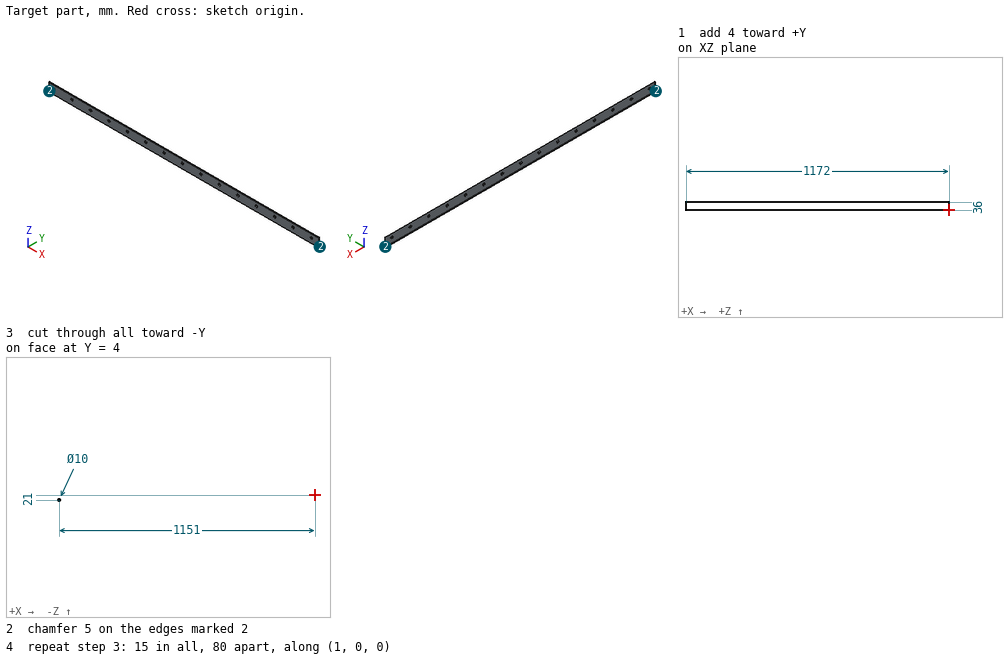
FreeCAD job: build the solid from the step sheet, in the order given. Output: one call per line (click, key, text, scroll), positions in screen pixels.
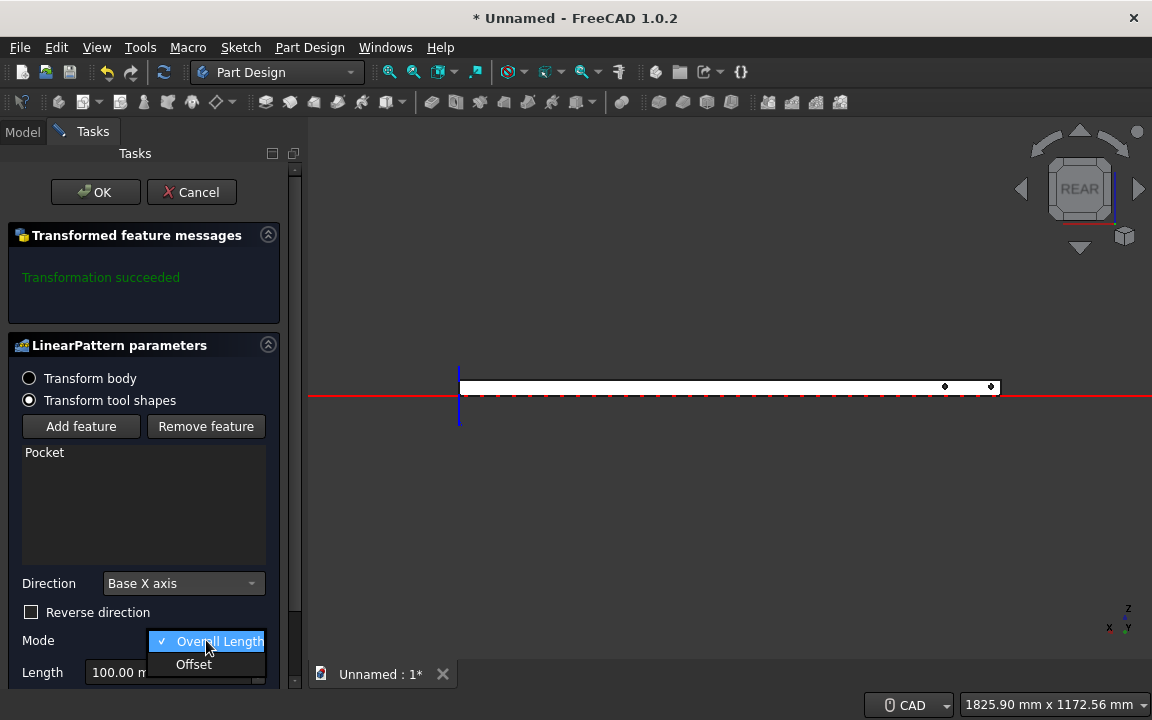
click(206, 664)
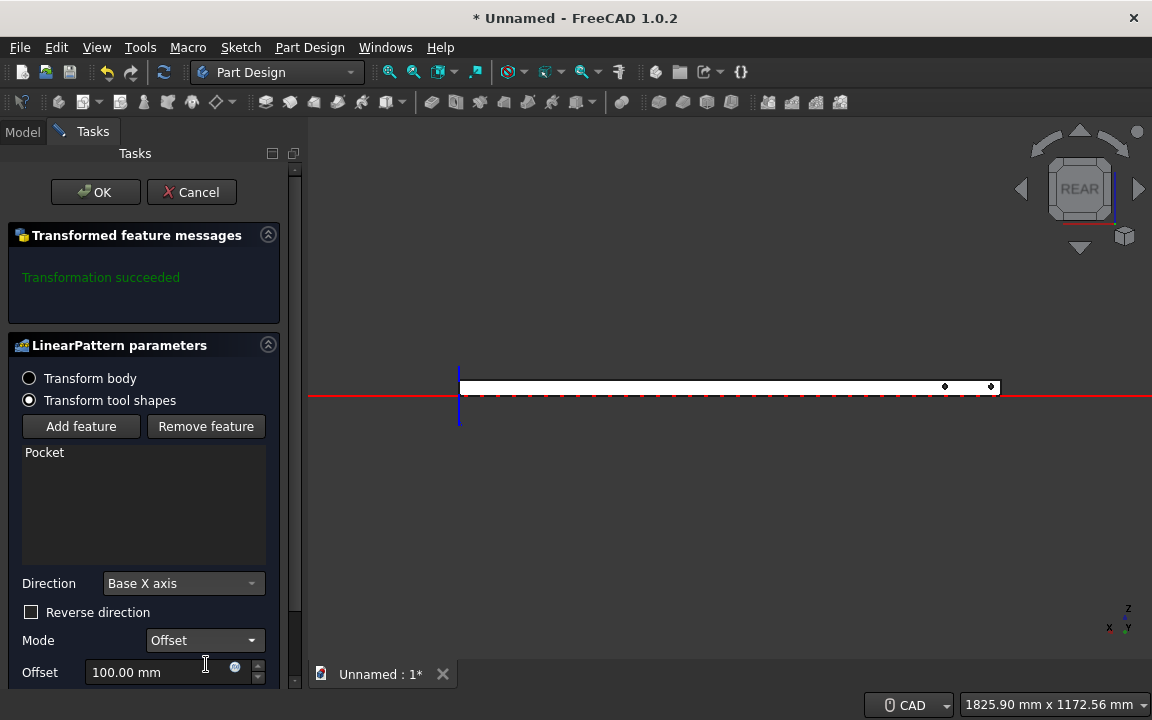
triple_click(168, 672)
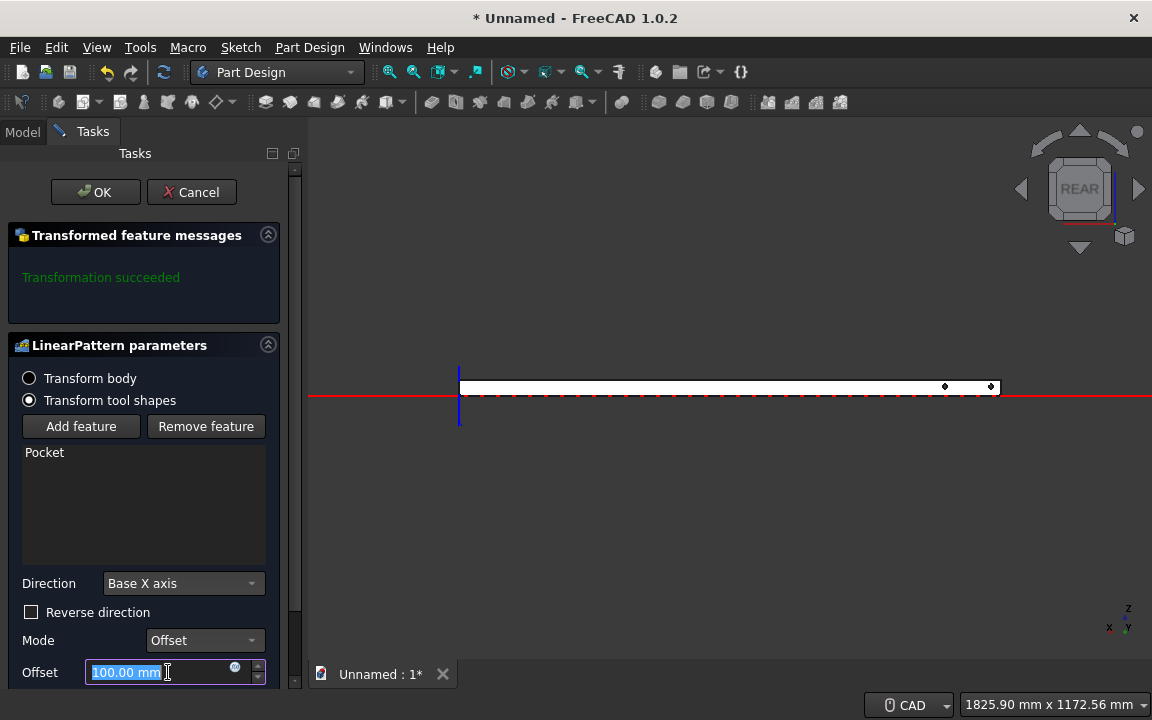
text(80)
key(Tab)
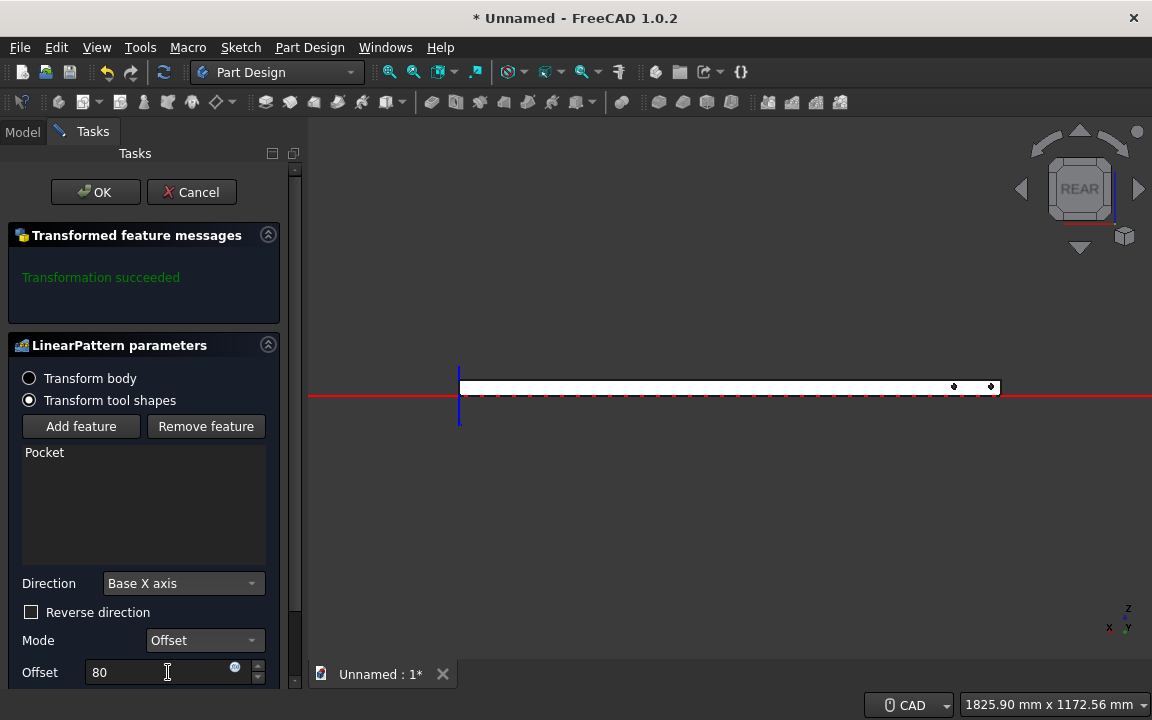
scroll(295, 426, down, 2)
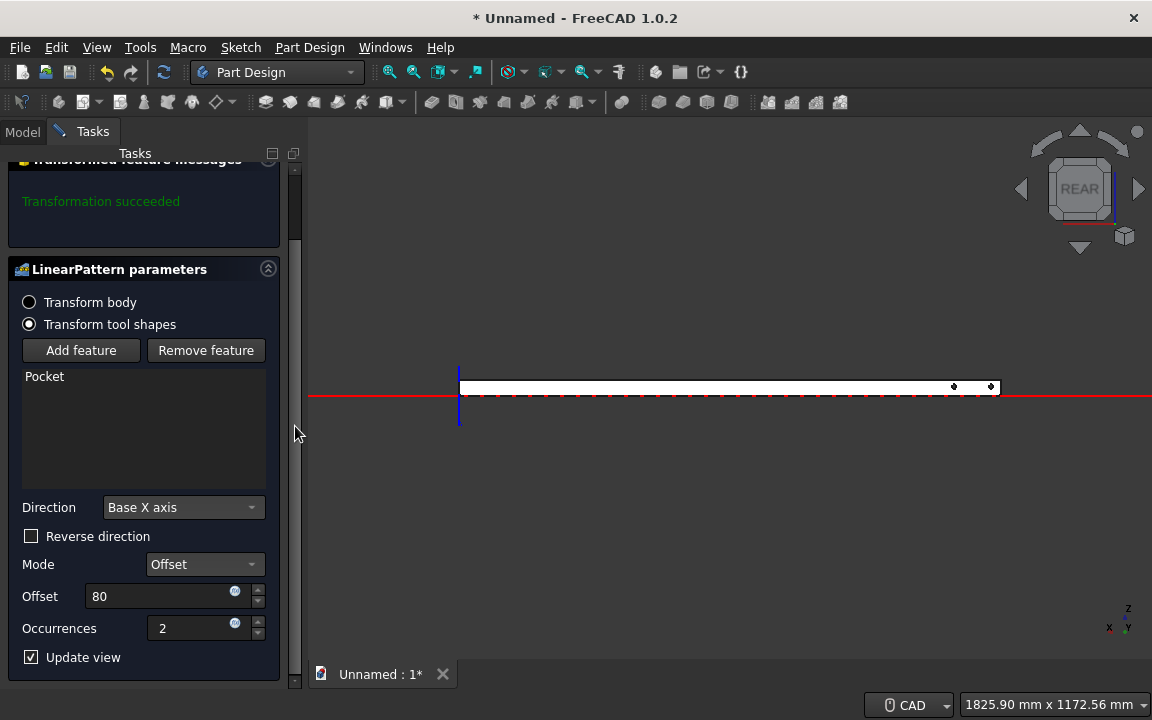
triple_click(198, 628)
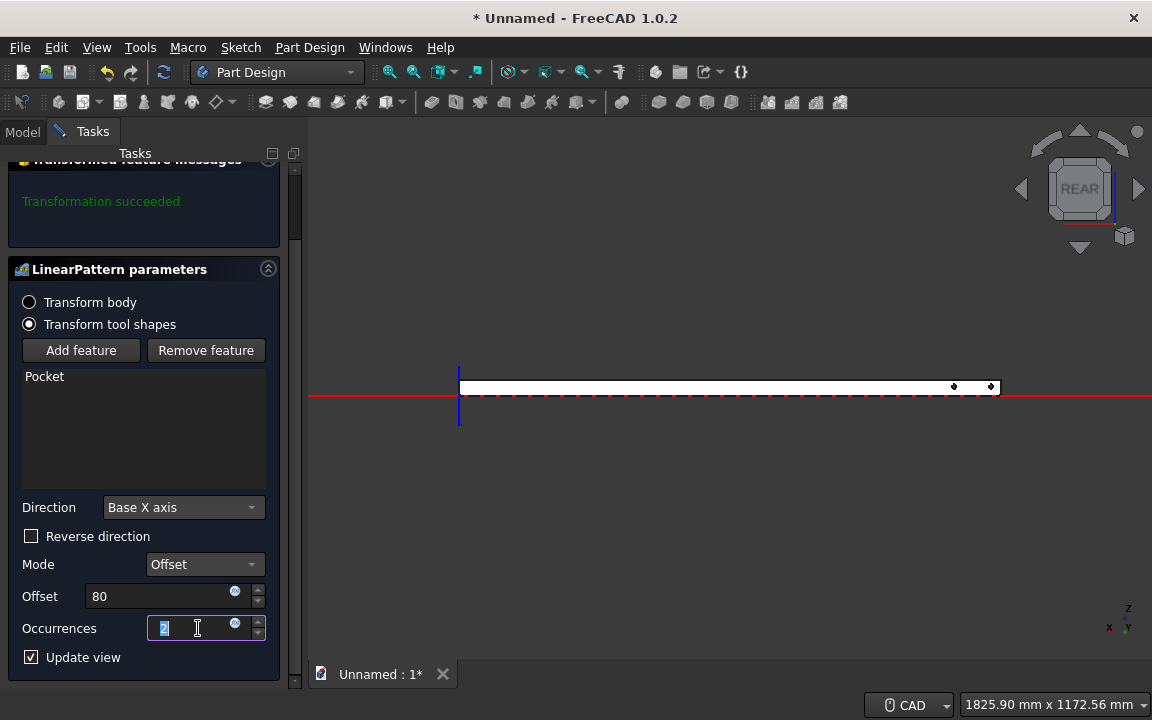
text(15)
key(Tab)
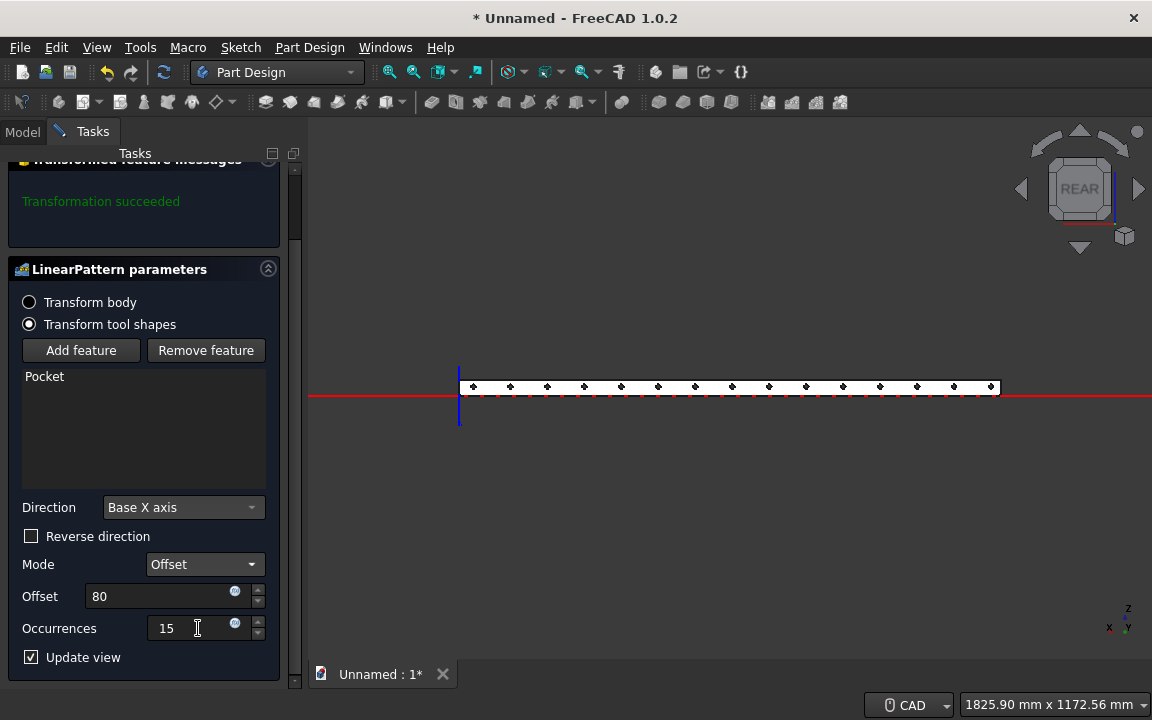
scroll(295, 426, up, 3)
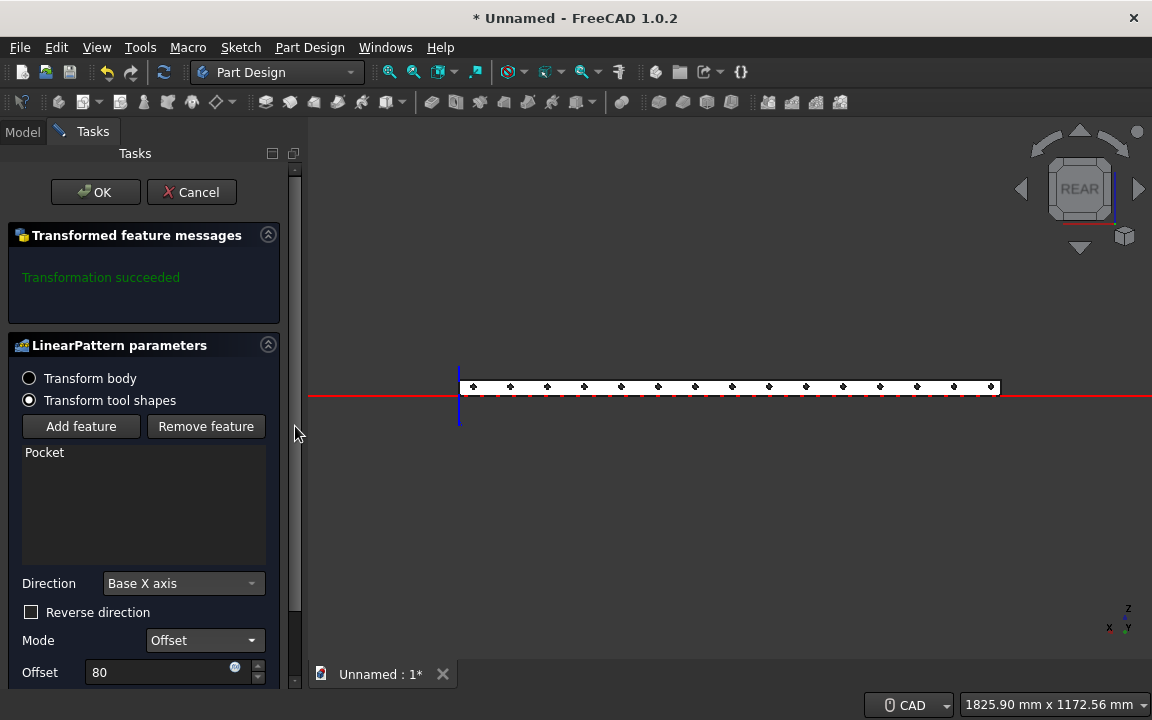
click(96, 192)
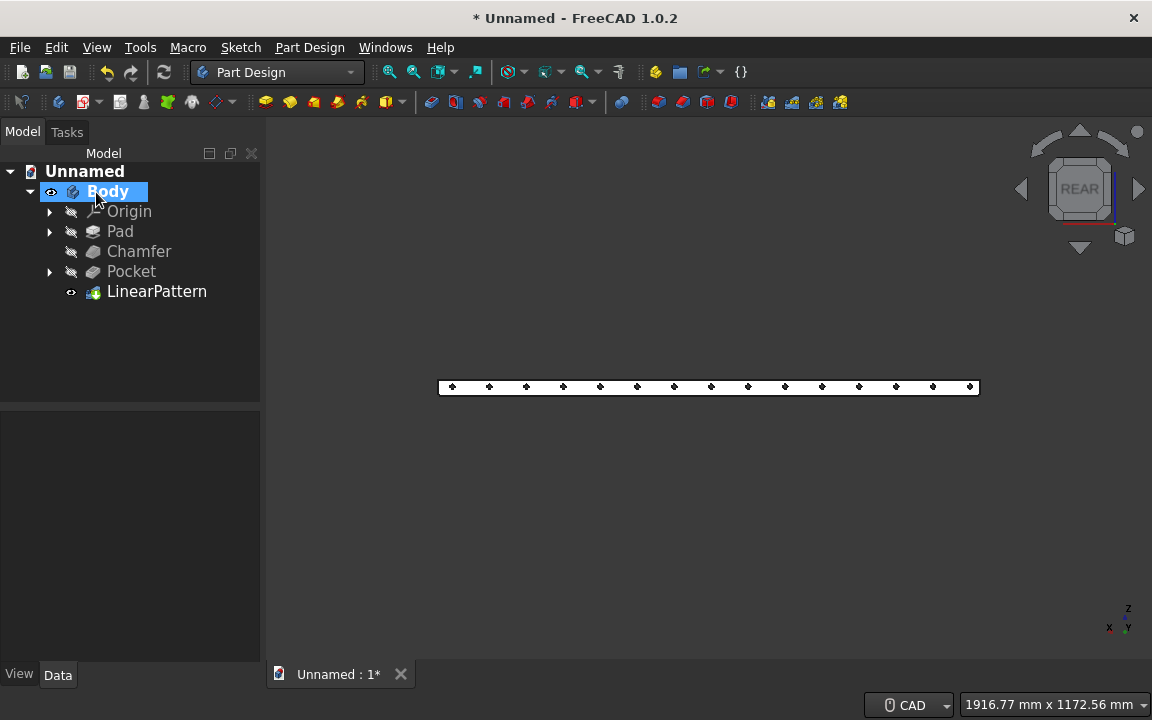
key(0)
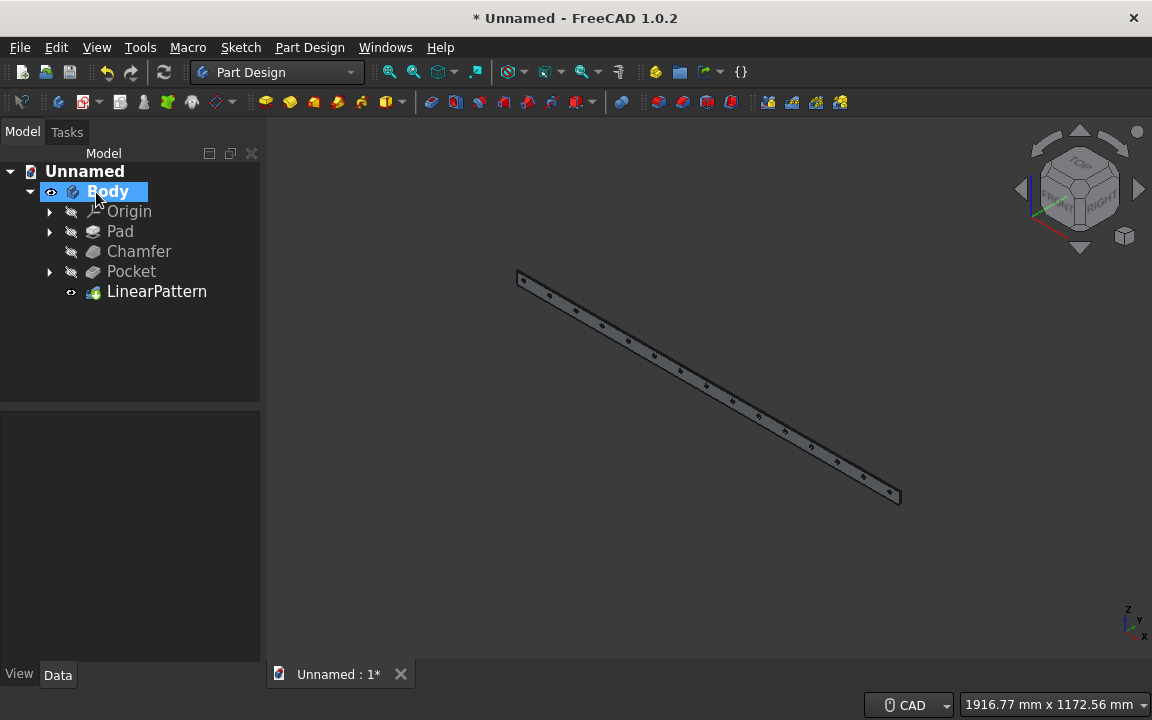
click(390, 72)